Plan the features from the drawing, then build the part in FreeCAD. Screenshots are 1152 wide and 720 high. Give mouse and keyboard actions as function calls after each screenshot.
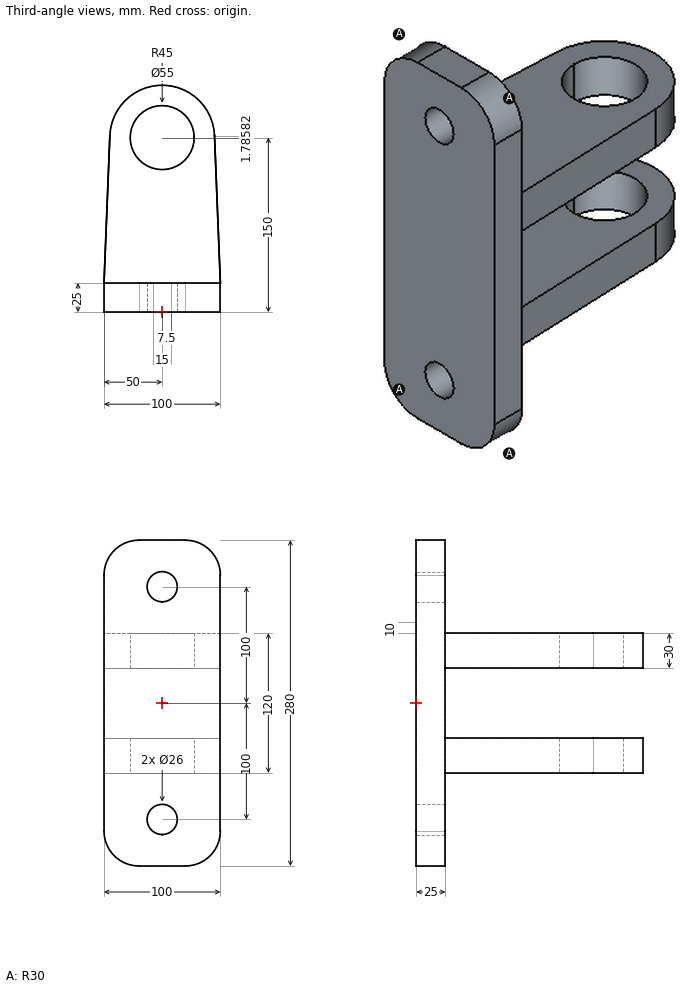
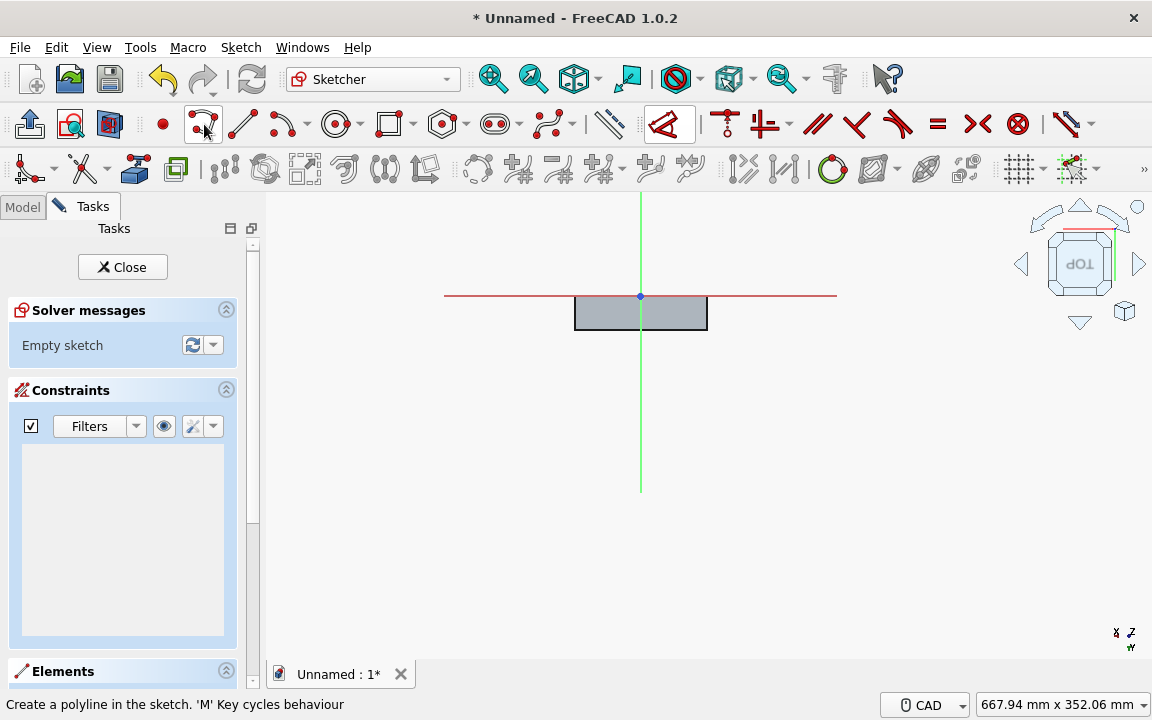
click(701, 498)
click(710, 330)
click(575, 330)
click(584, 498)
right_click(584, 498)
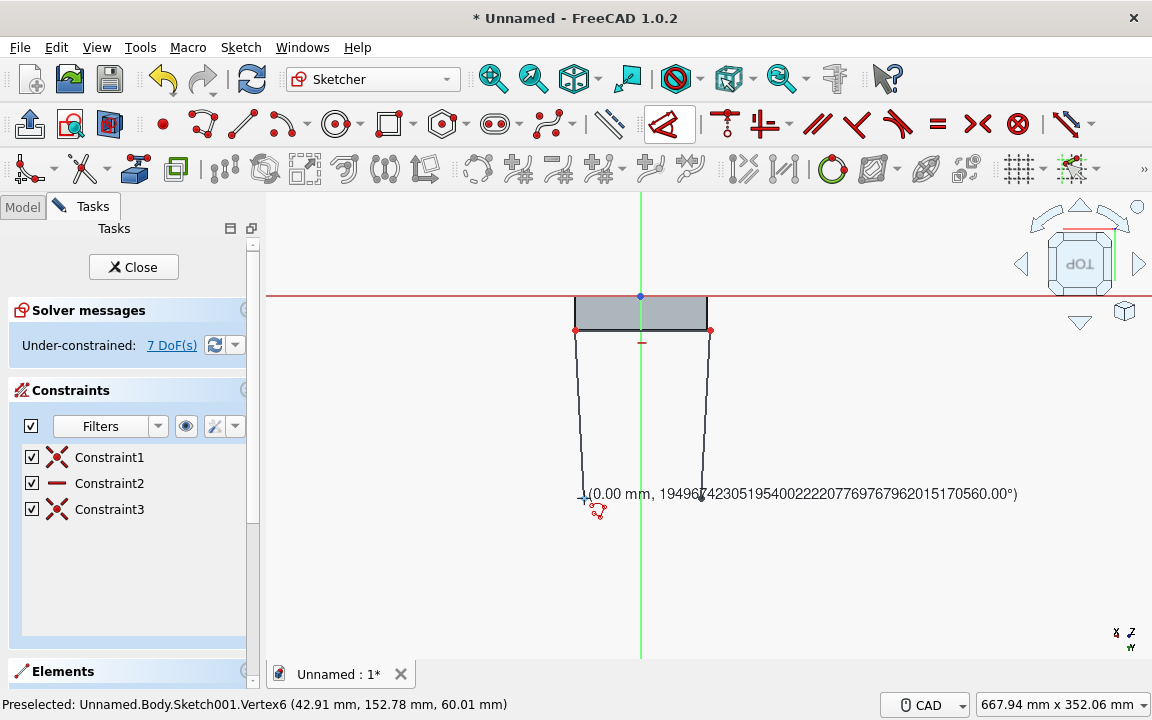
key(g)
key(3)
key(a)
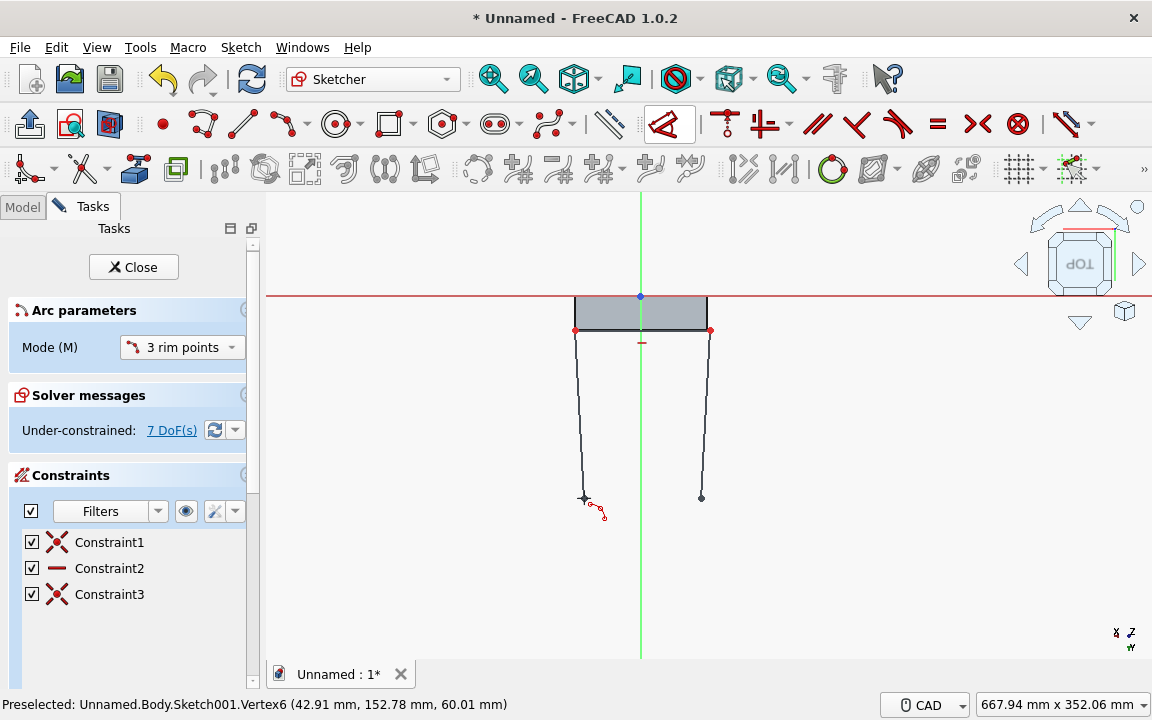
click(584, 499)
click(701, 499)
click(623, 552)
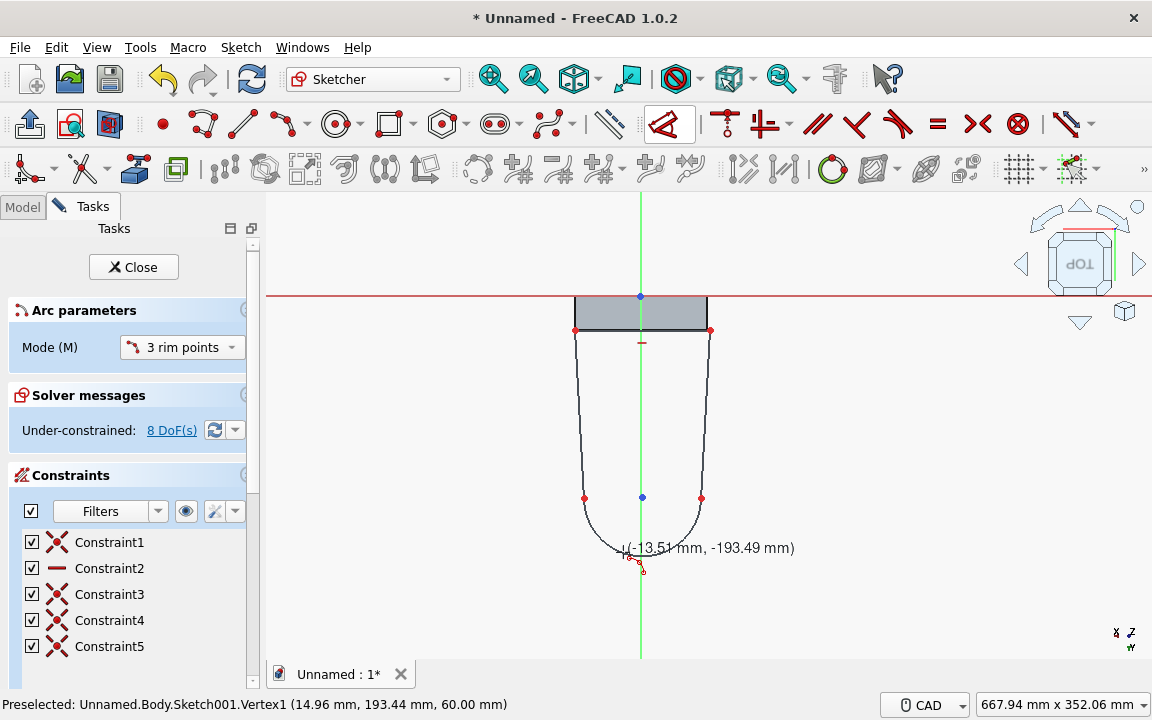
click(336, 124)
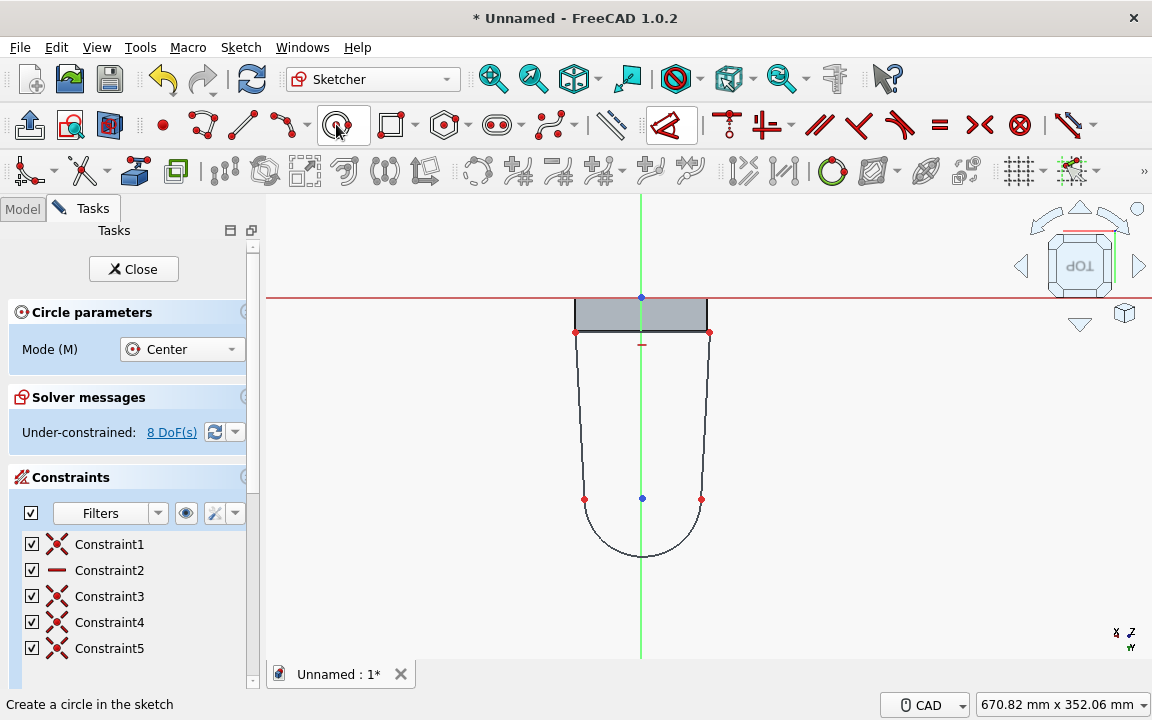
click(641, 496)
click(667, 470)
key(Escape)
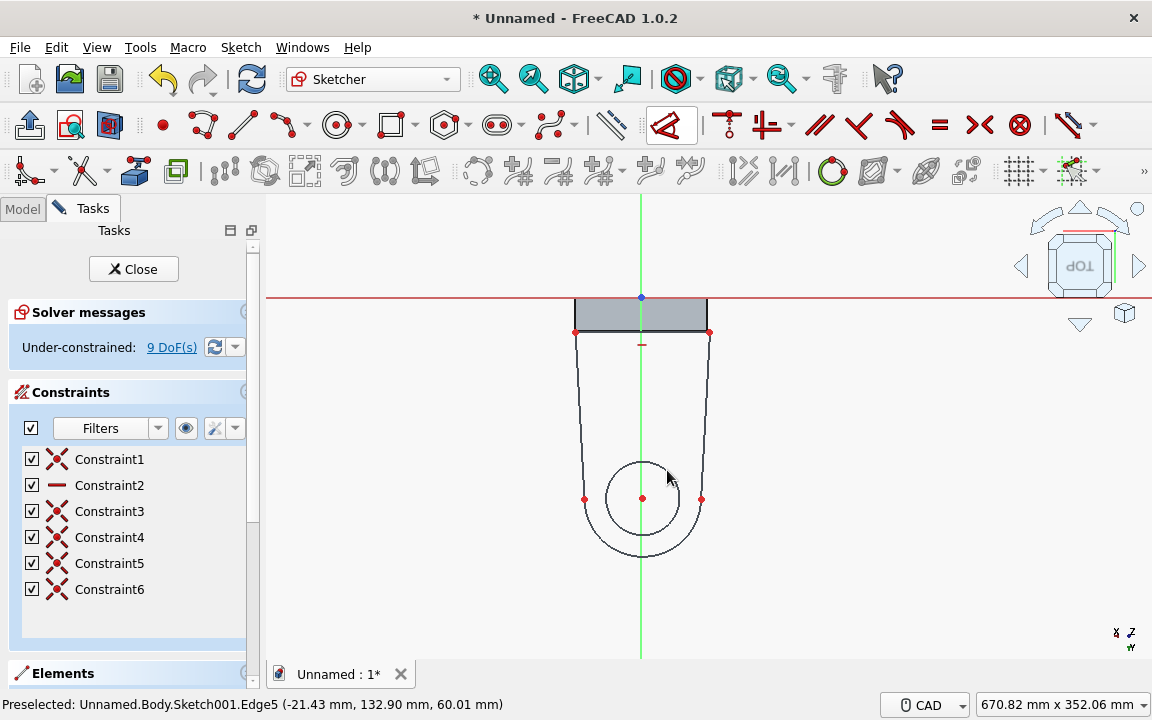
click(643, 499)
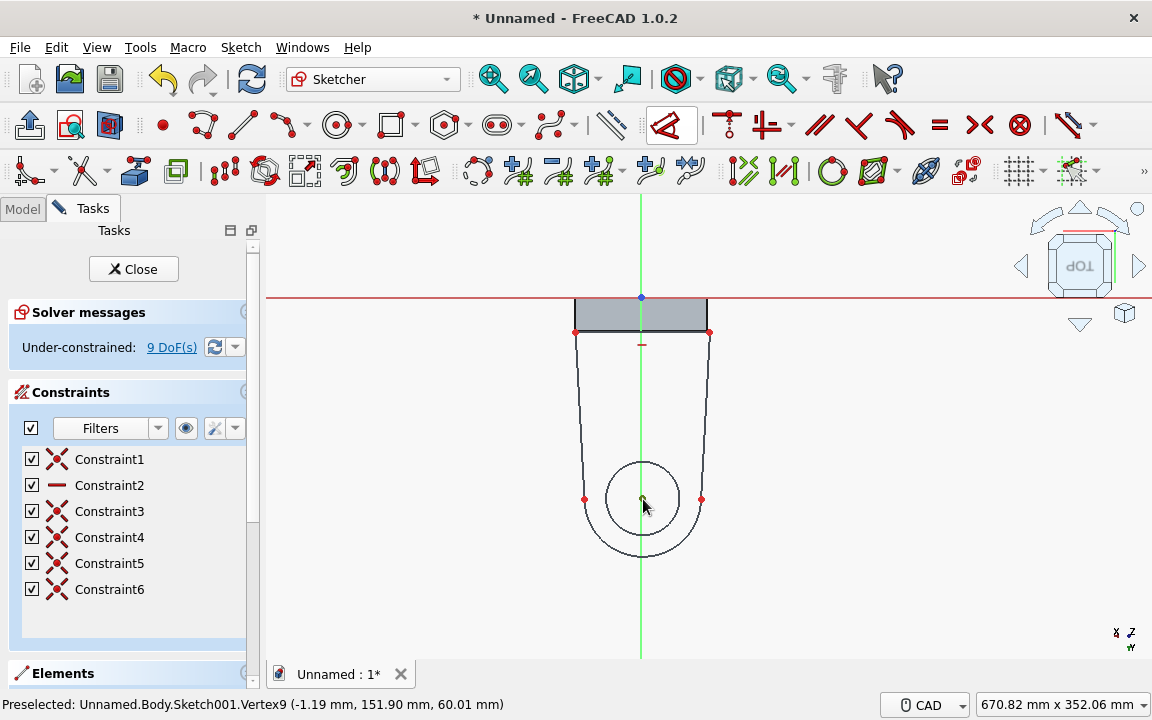
click(641, 602)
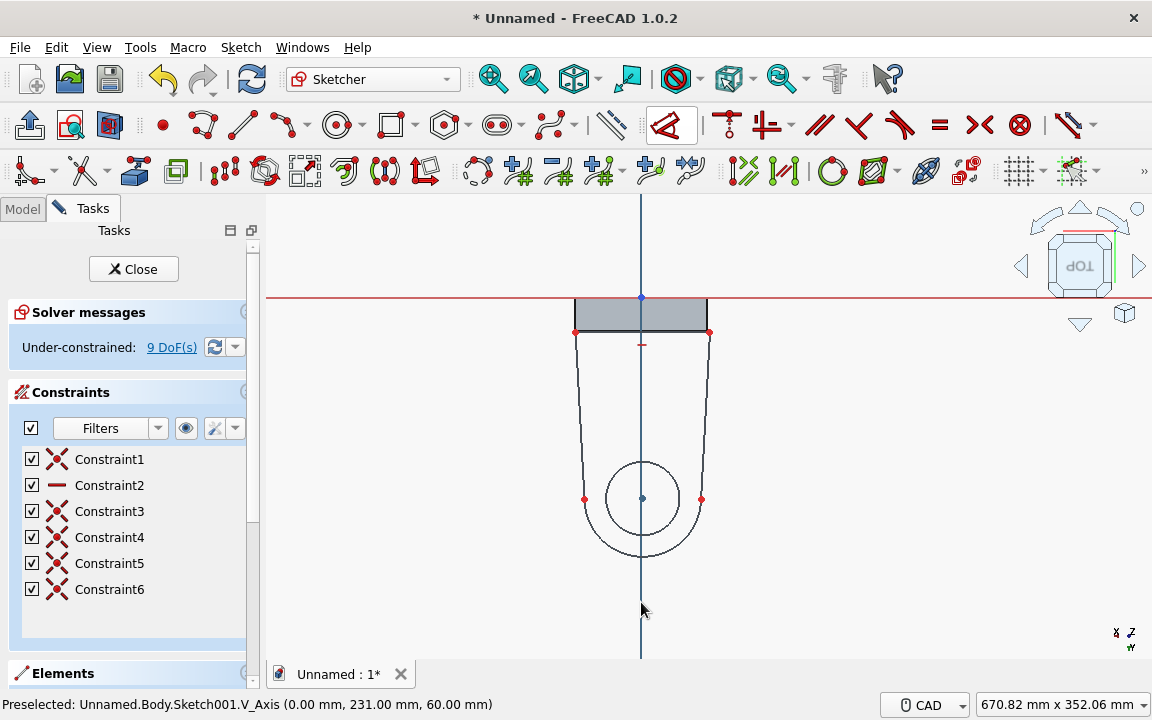
click(728, 126)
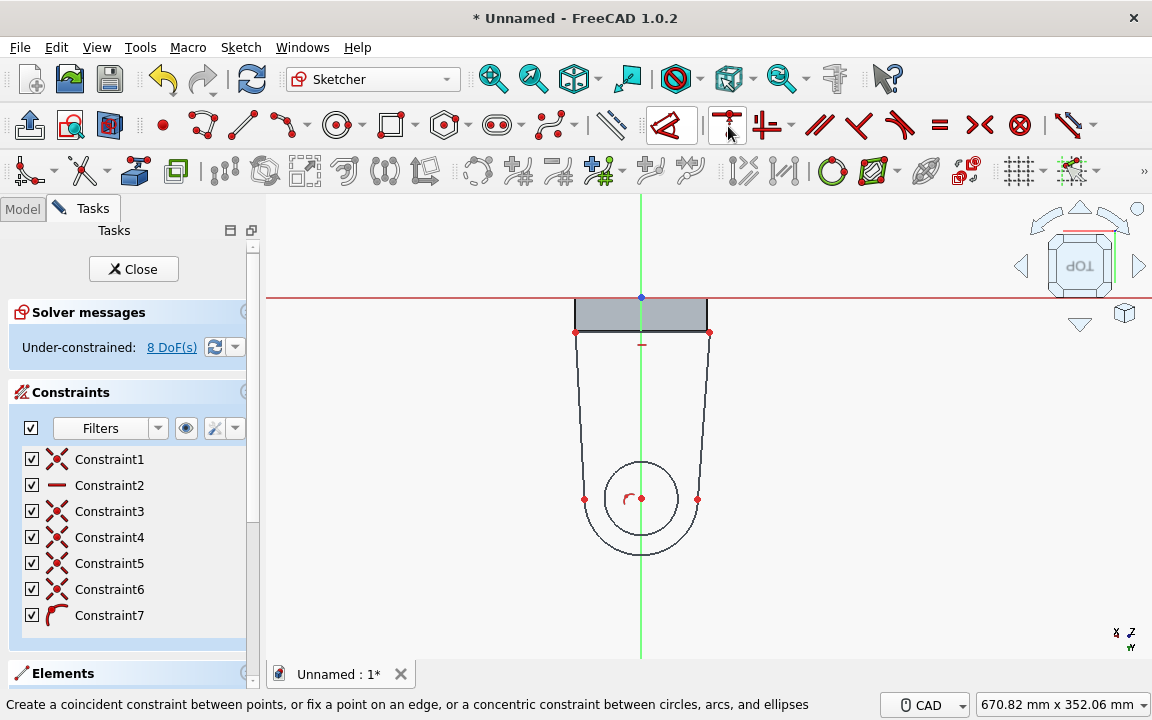
click(608, 545)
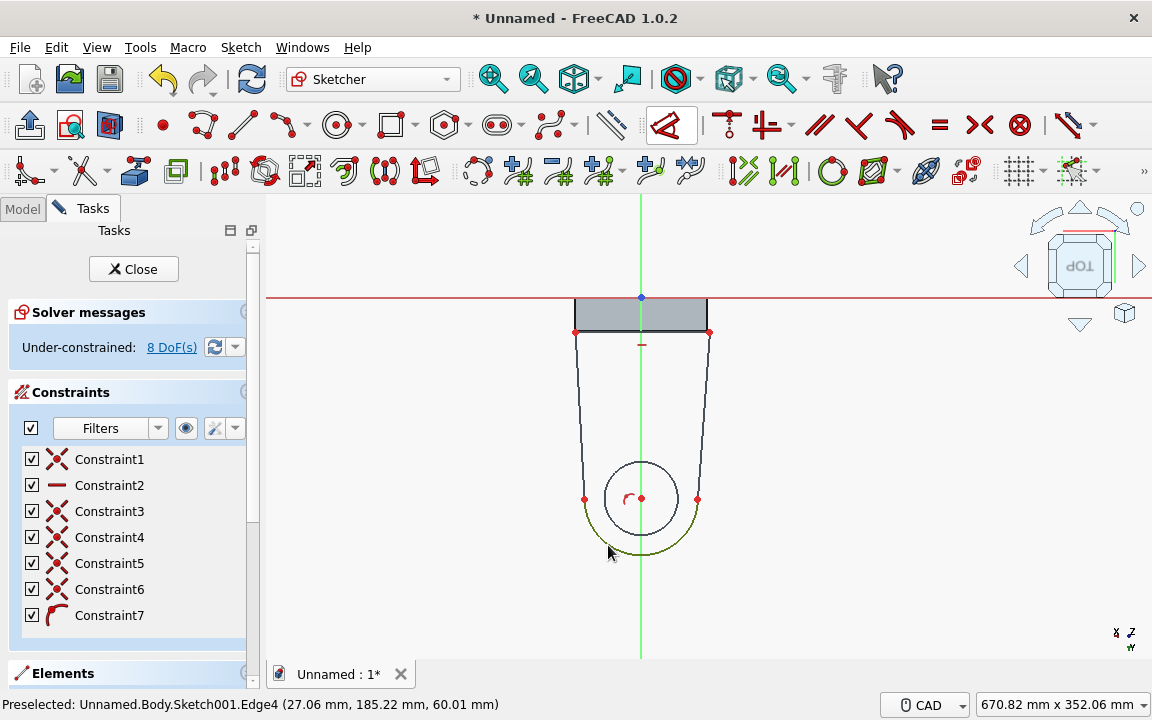
click(692, 126)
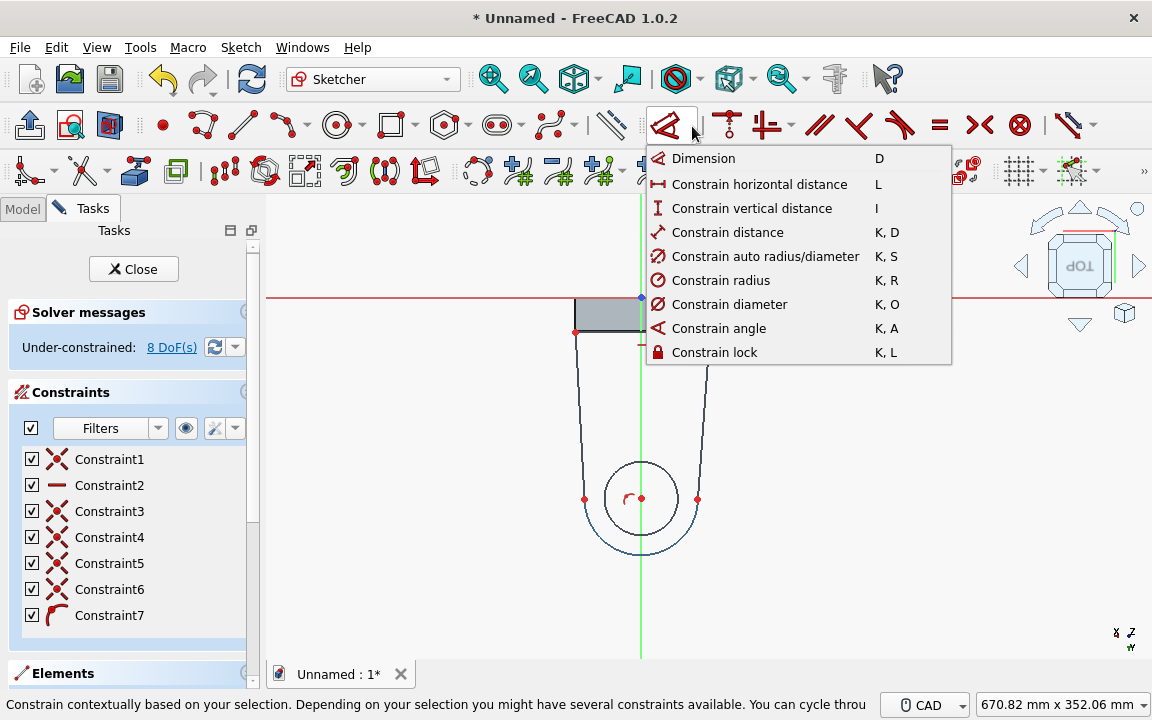
click(799, 280)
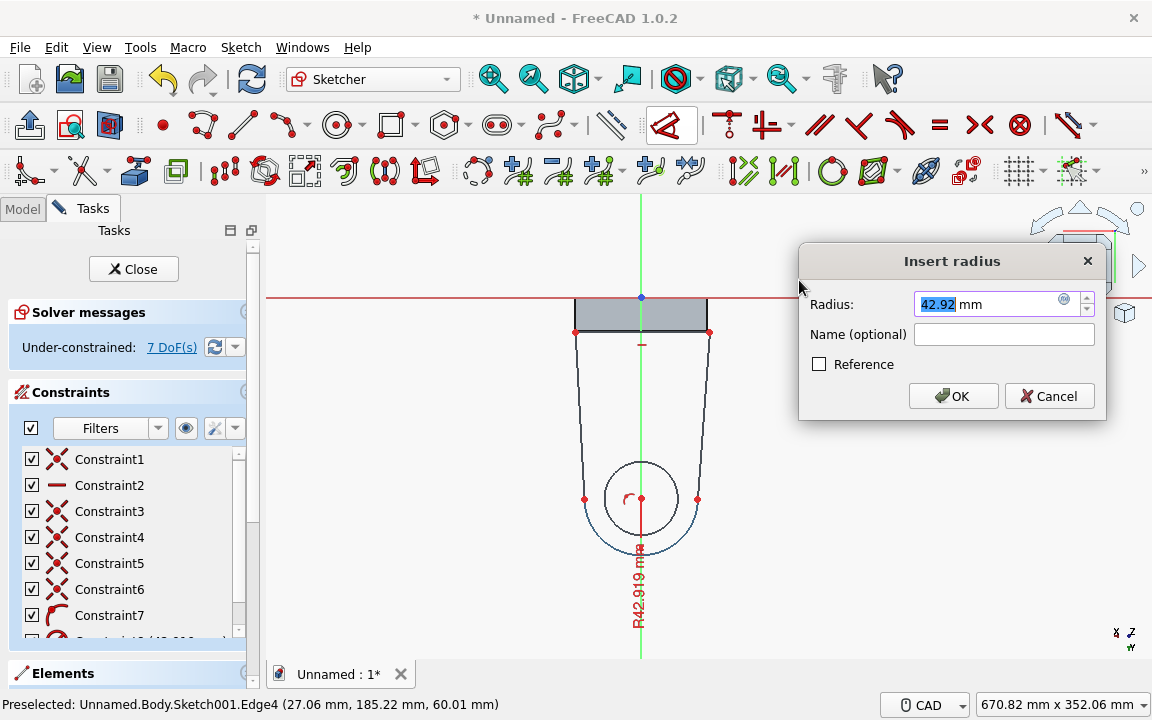
text(45)
key(Return)